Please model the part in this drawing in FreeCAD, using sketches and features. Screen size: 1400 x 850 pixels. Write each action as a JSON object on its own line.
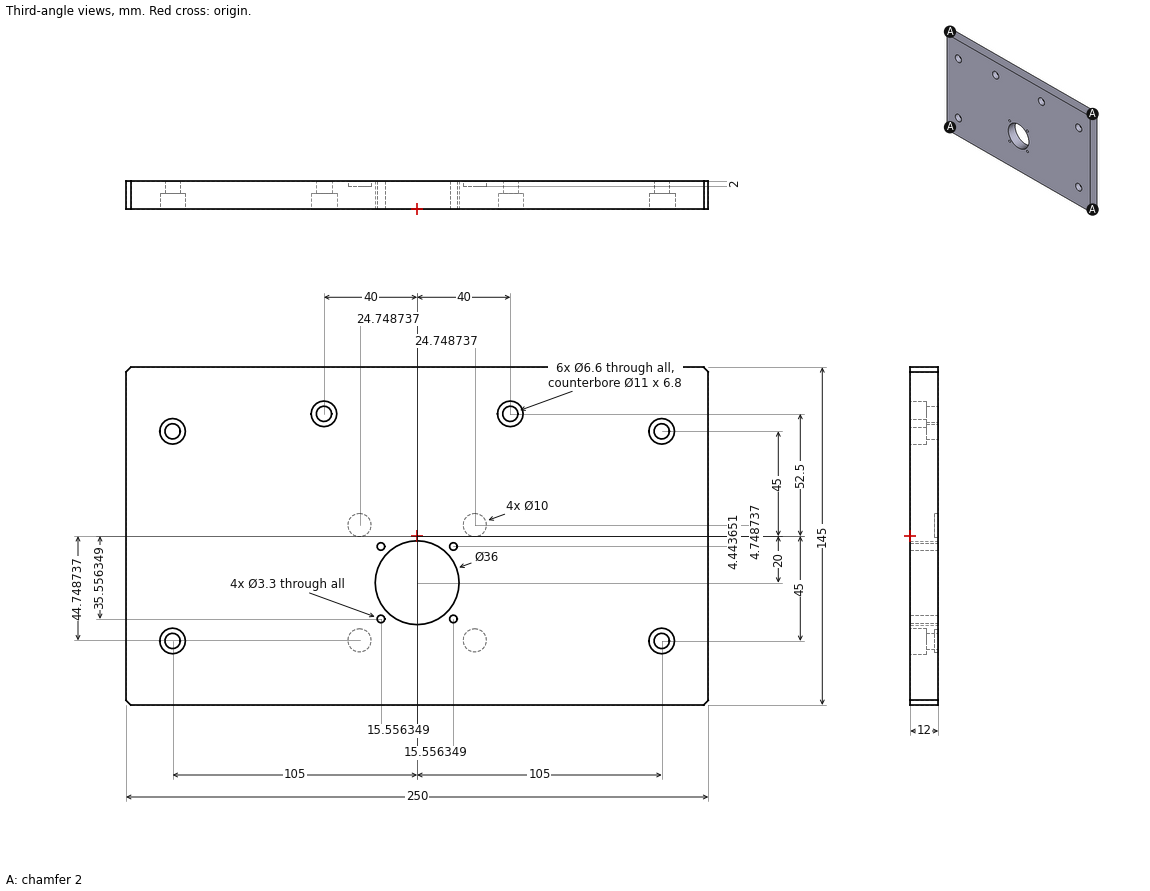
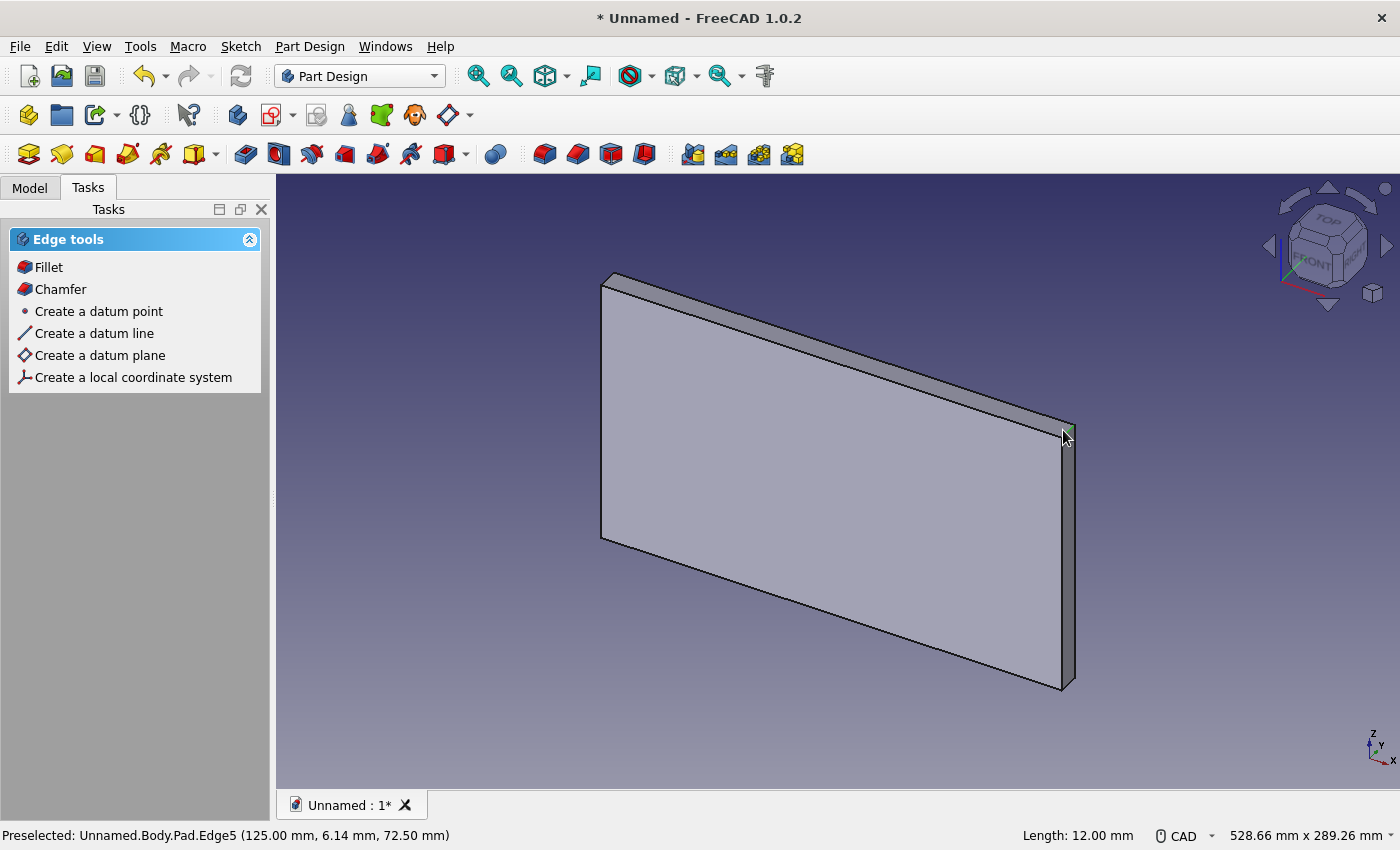
{"action": "key", "text": "0"}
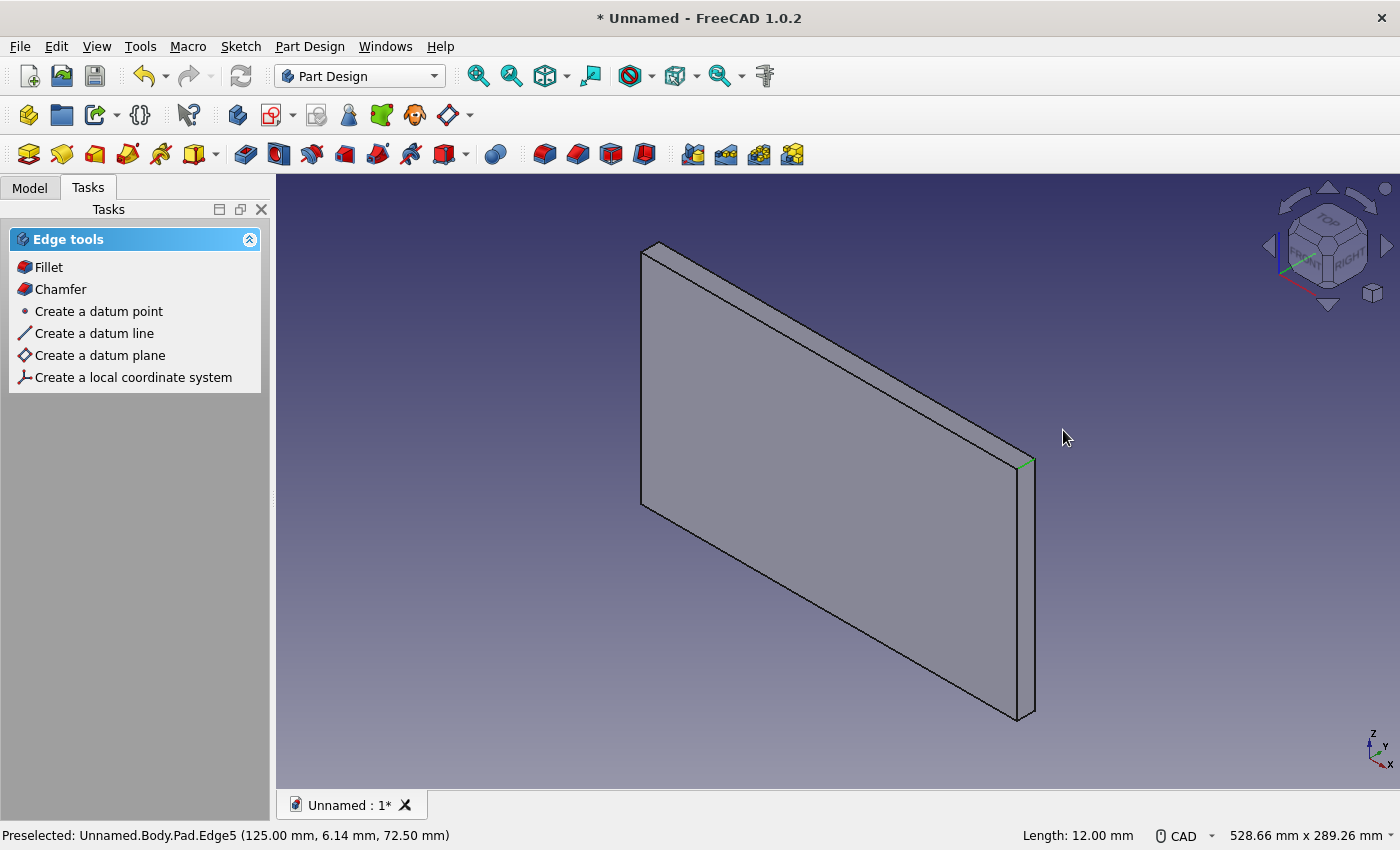
{"action": "key", "text": "2"}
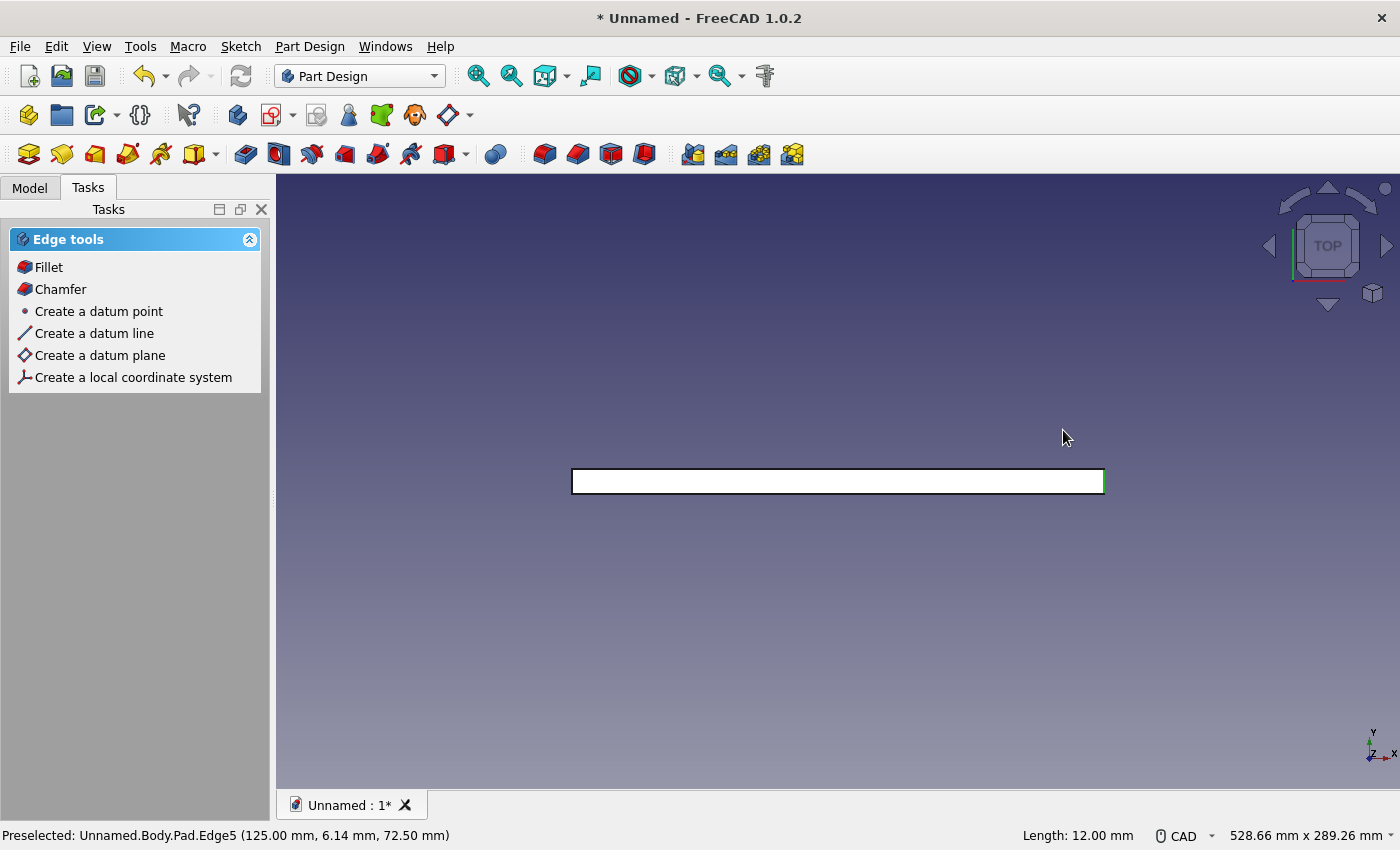
{"action": "left_click", "coordinate": [572, 480], "text": "ctrl"}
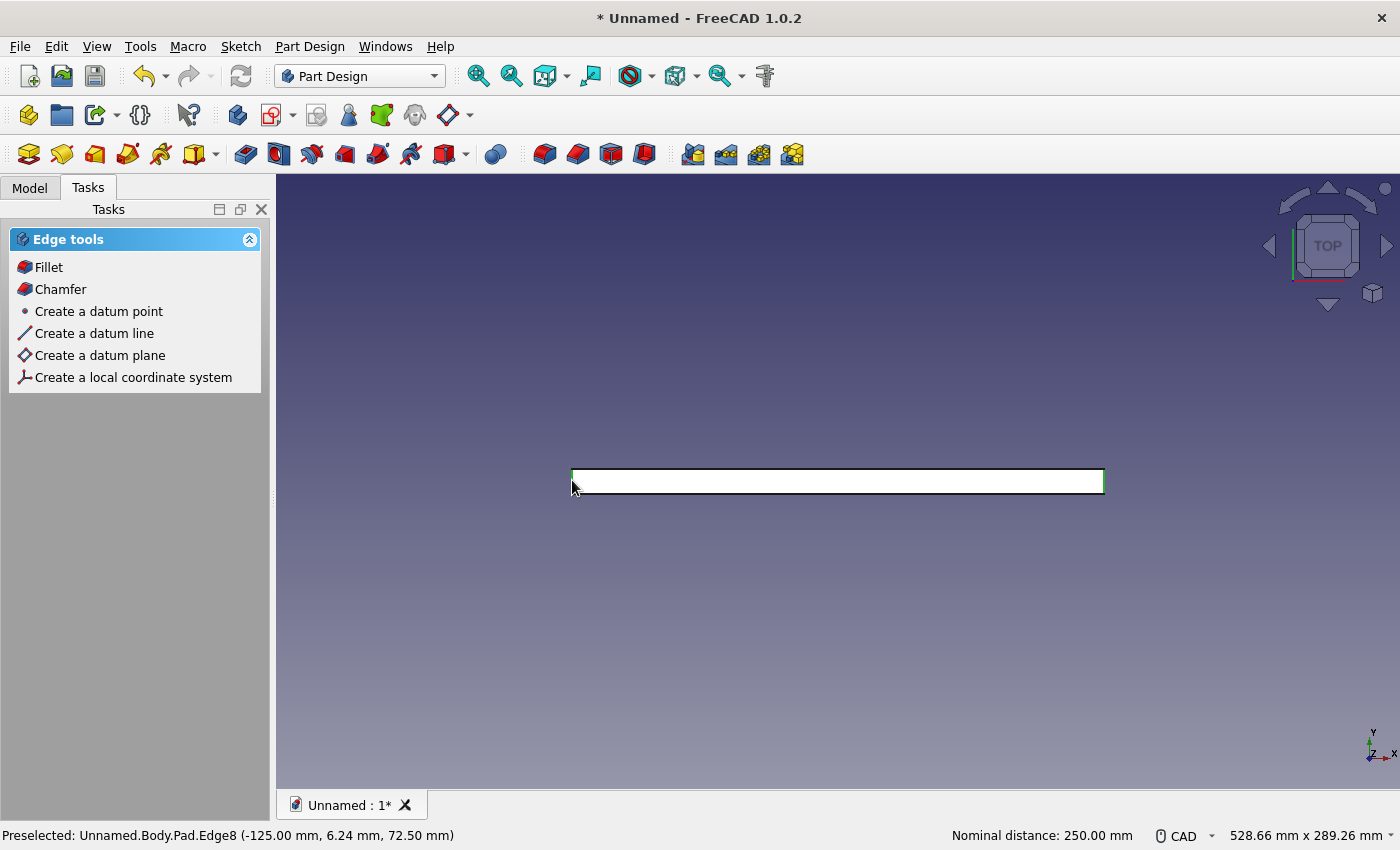
{"action": "key", "text": "1"}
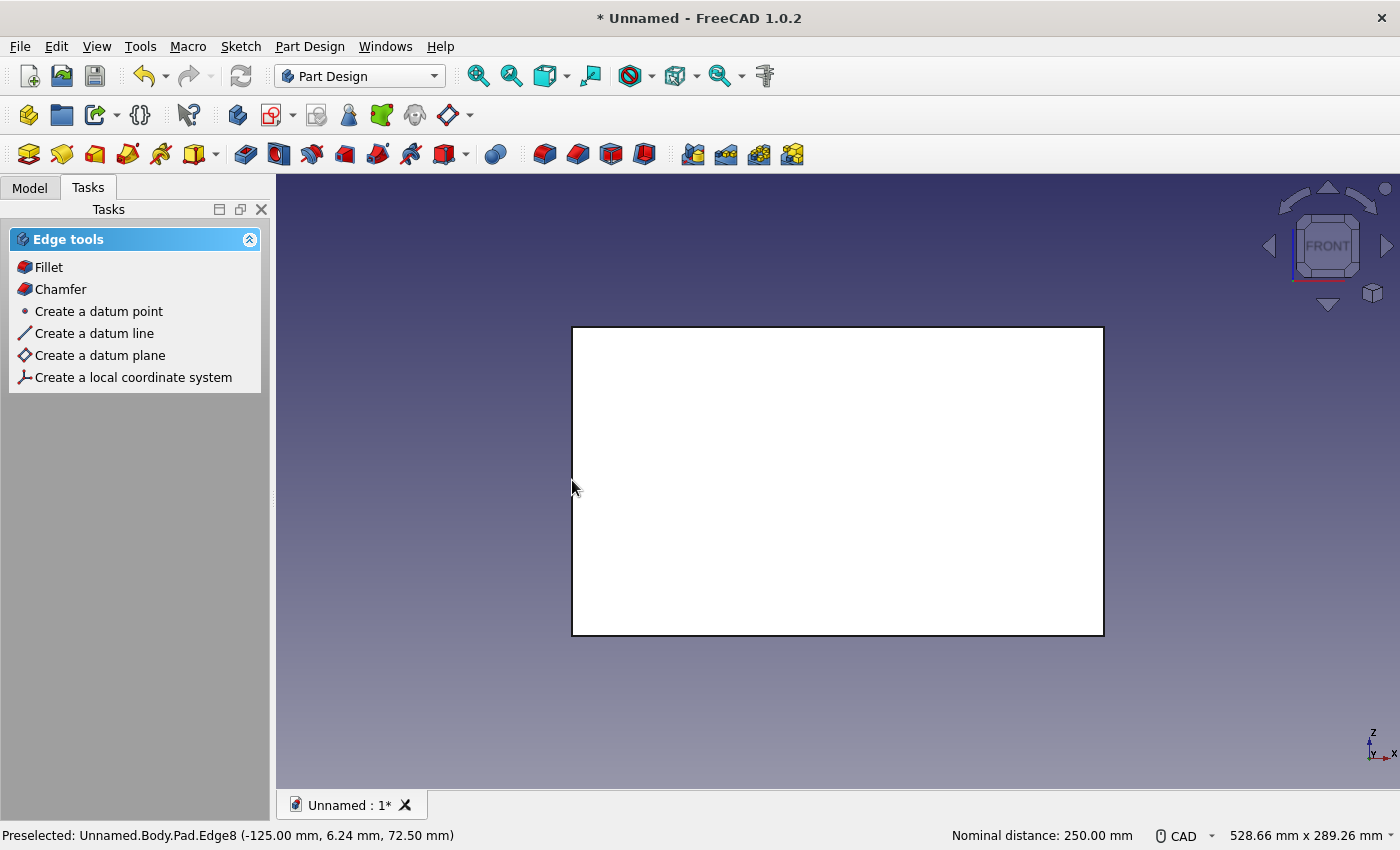
{"action": "key", "text": "3"}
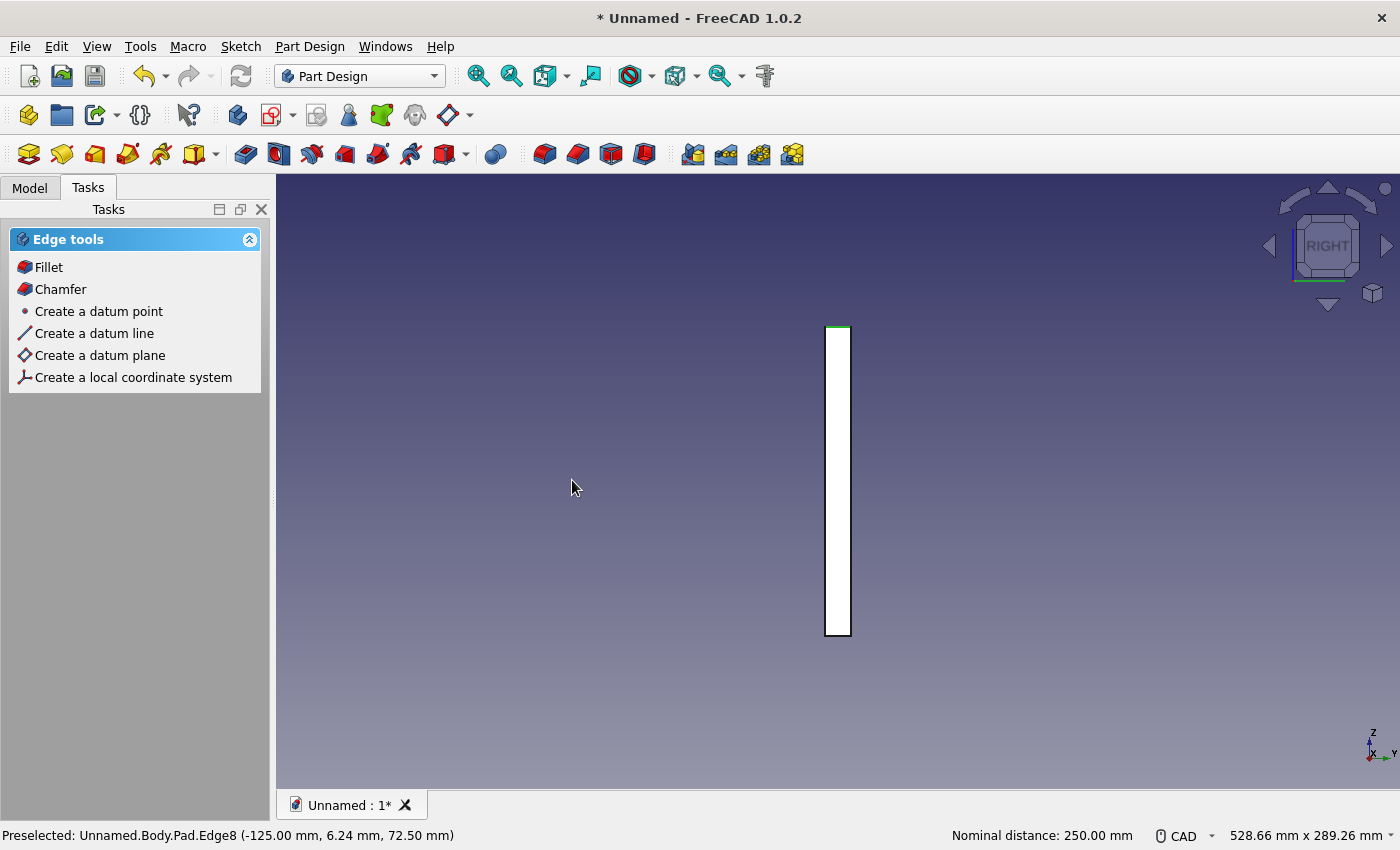
{"action": "left_click", "coordinate": [838, 635], "text": "ctrl"}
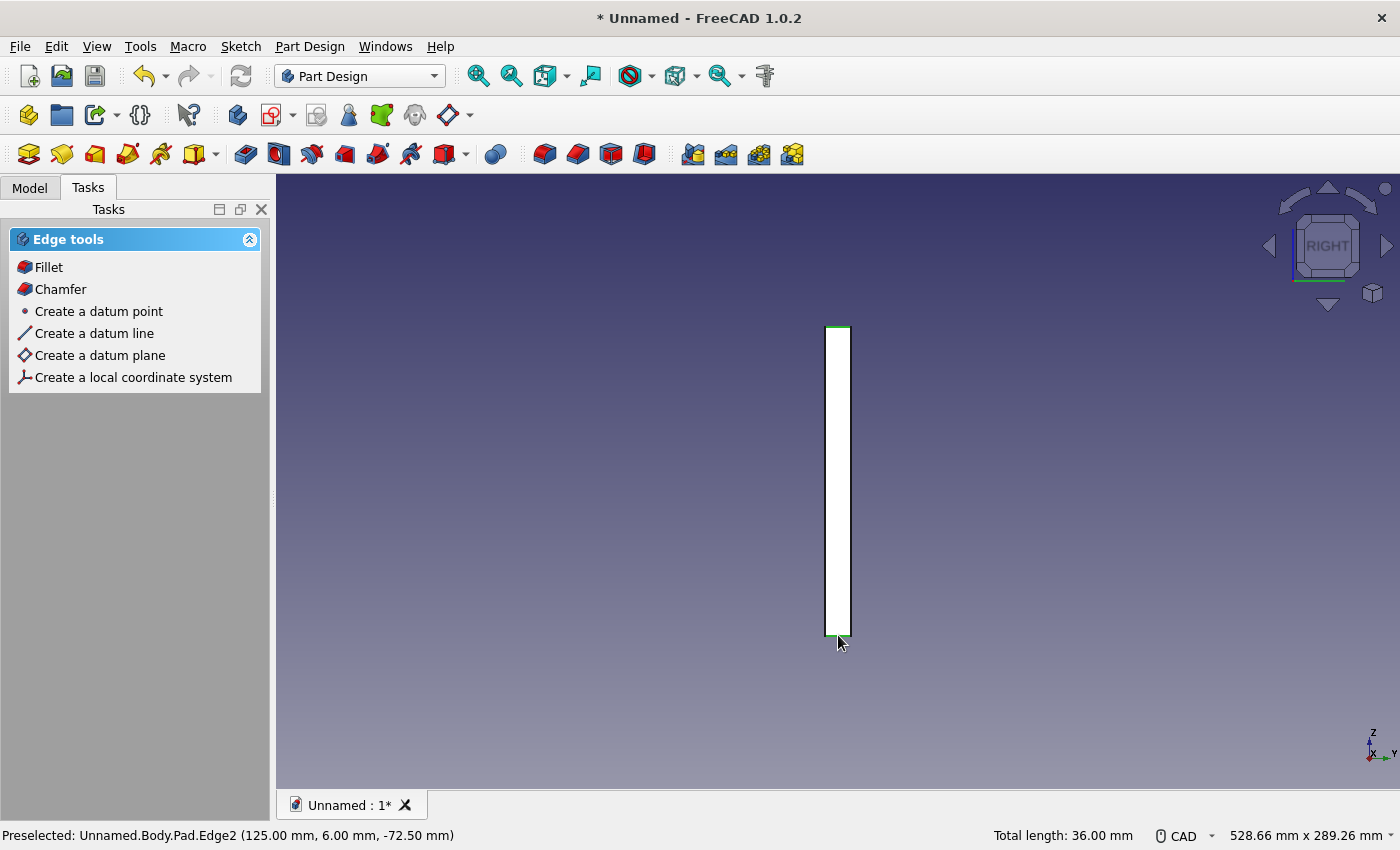
{"action": "key", "text": "5"}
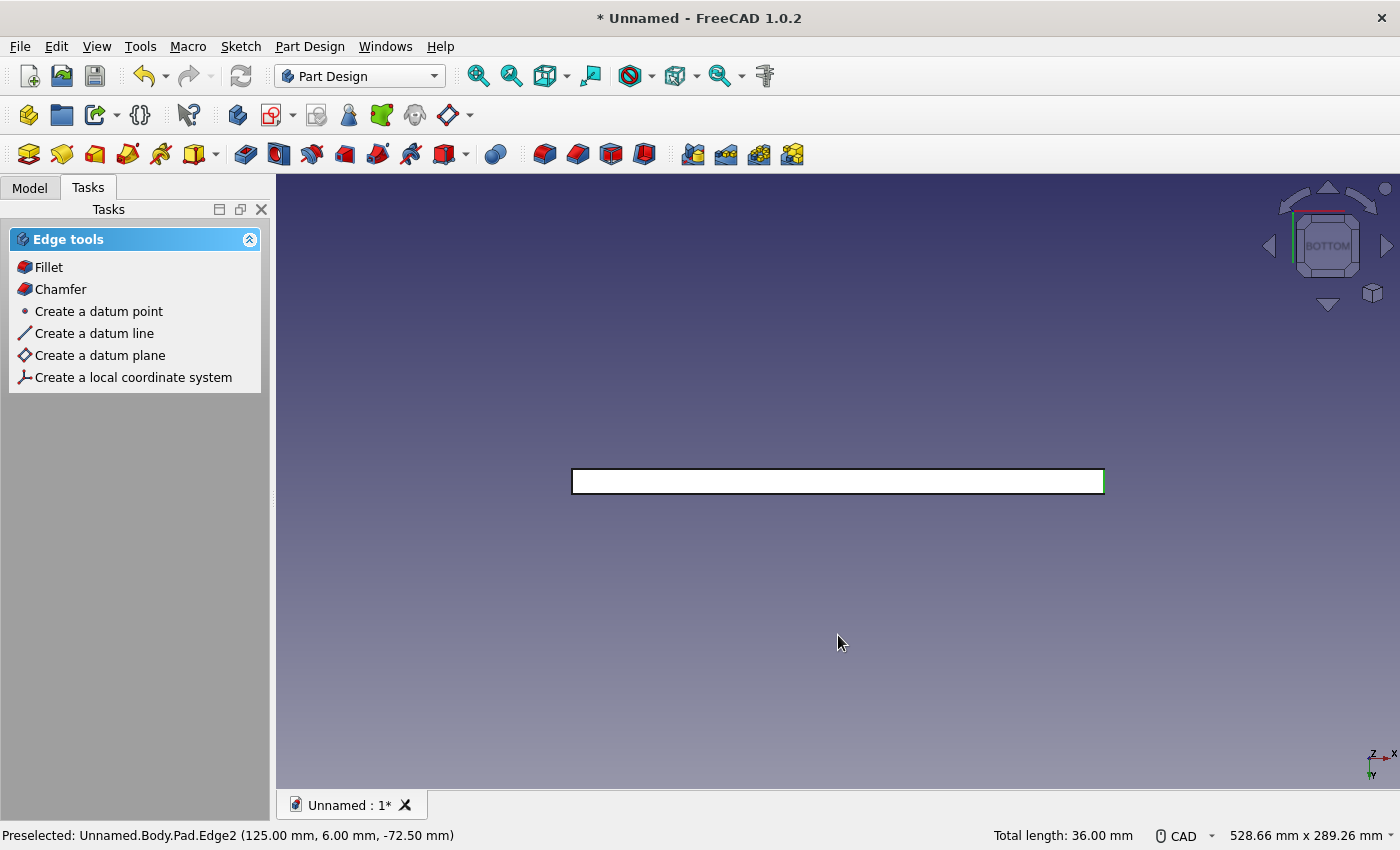
{"action": "left_click", "coordinate": [572, 480], "text": "ctrl"}